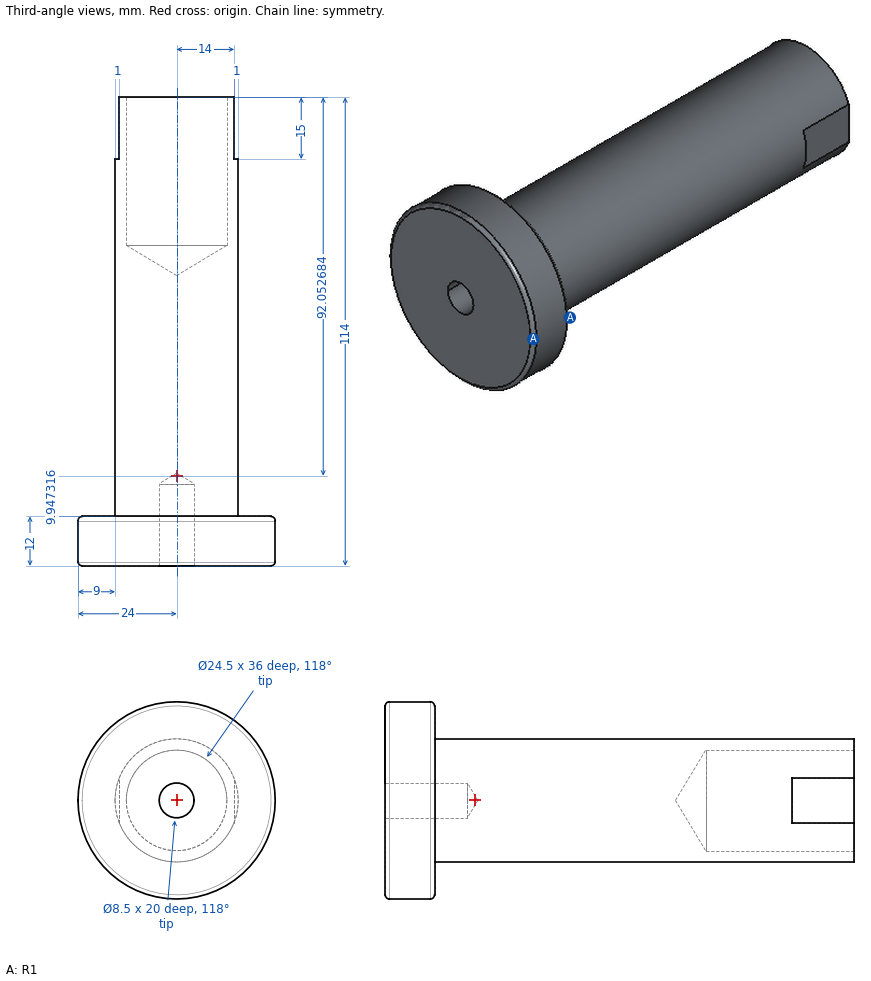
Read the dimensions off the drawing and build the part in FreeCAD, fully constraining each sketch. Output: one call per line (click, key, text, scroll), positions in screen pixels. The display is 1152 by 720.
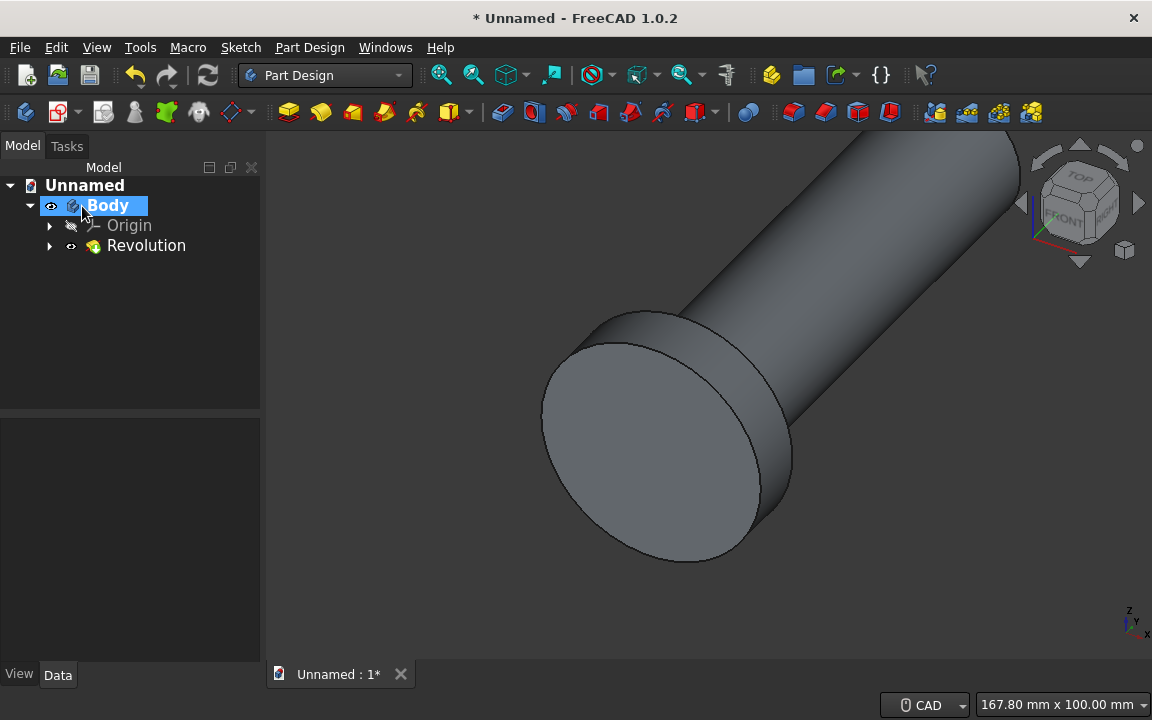
key(v)
key(f)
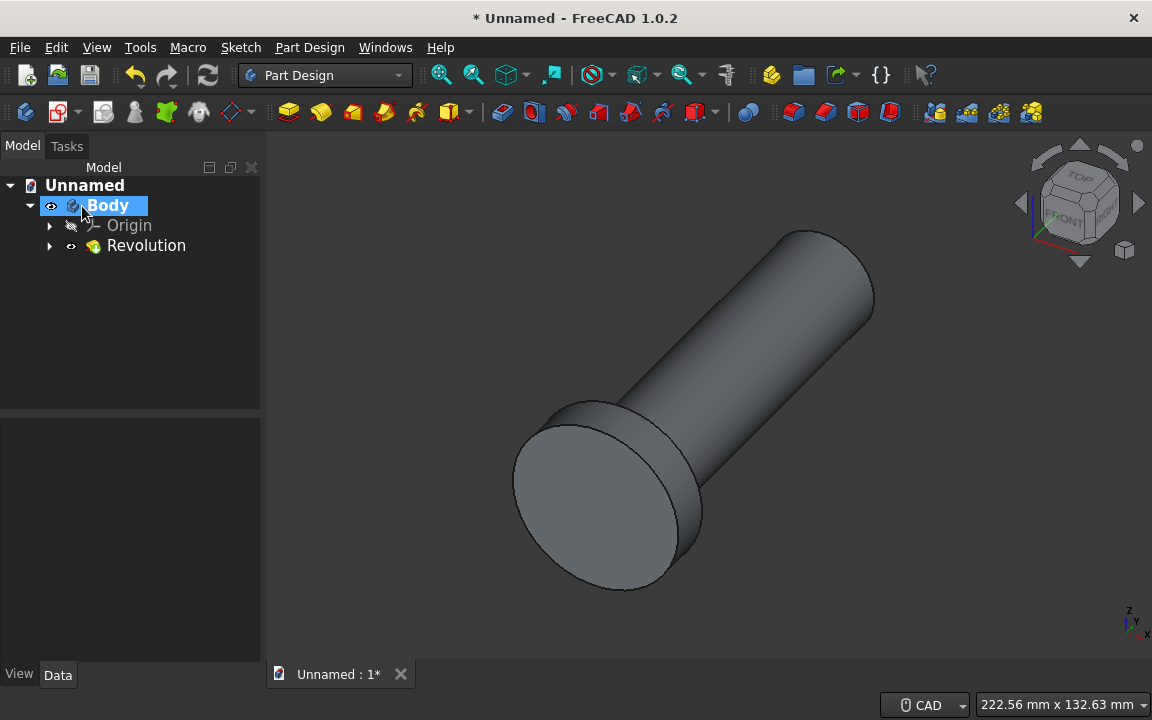
click(58, 112)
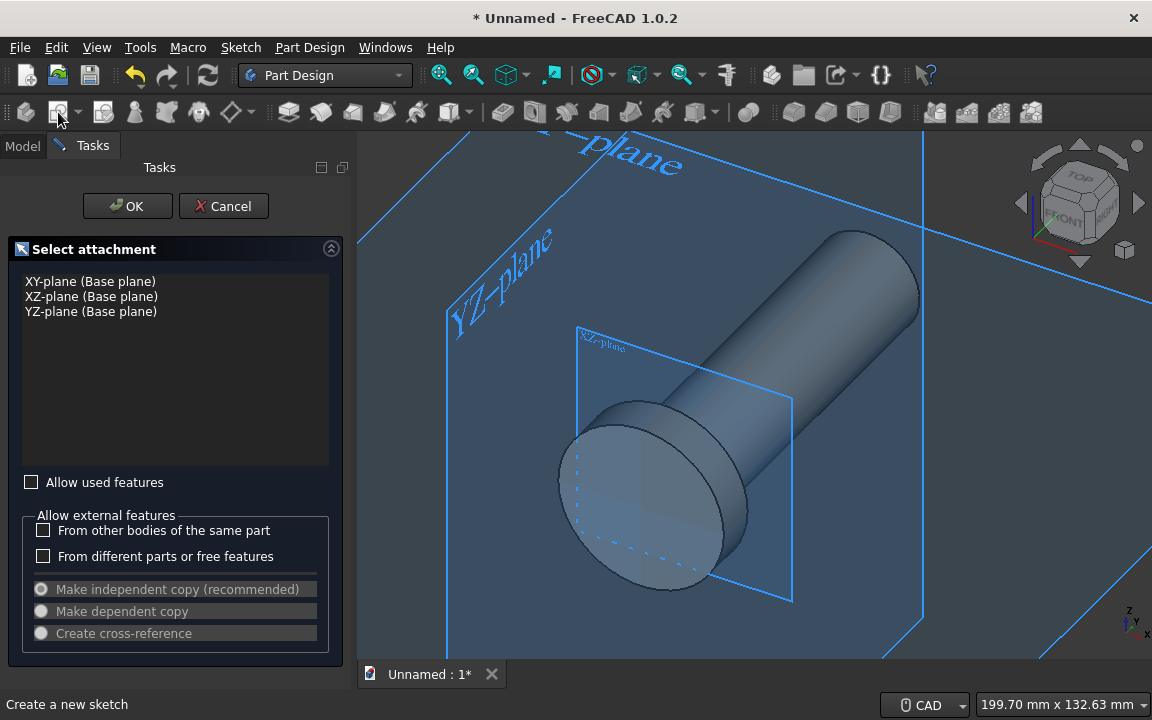
click(82, 282)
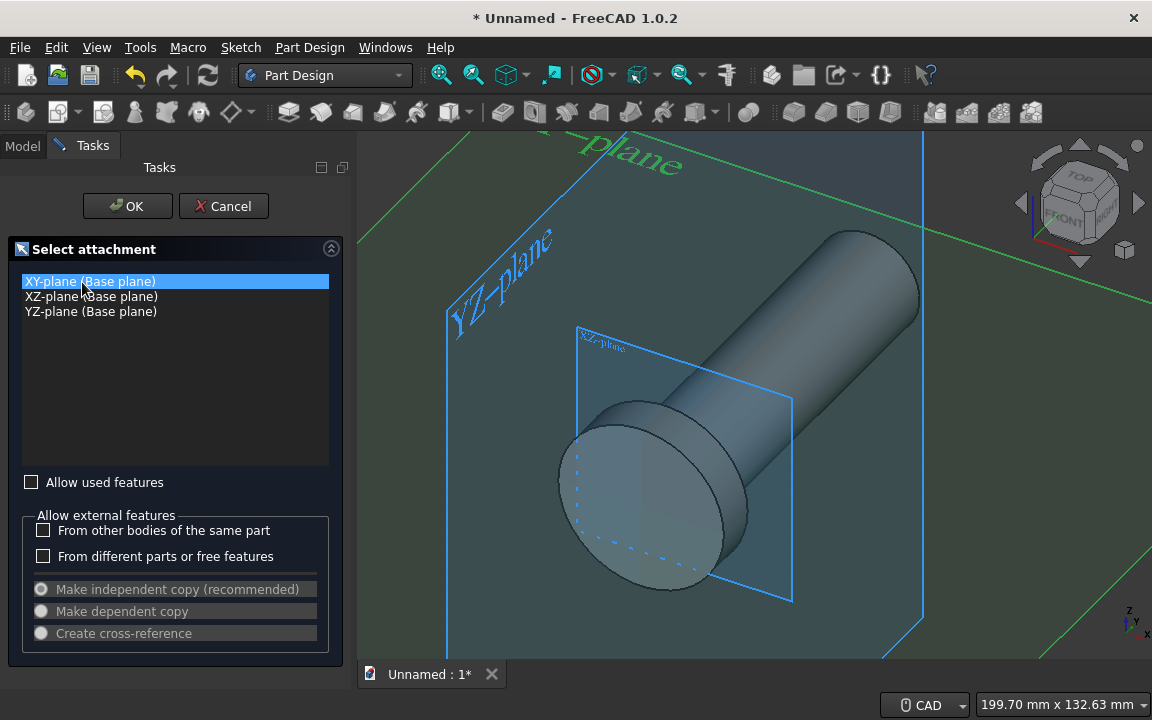
click(128, 206)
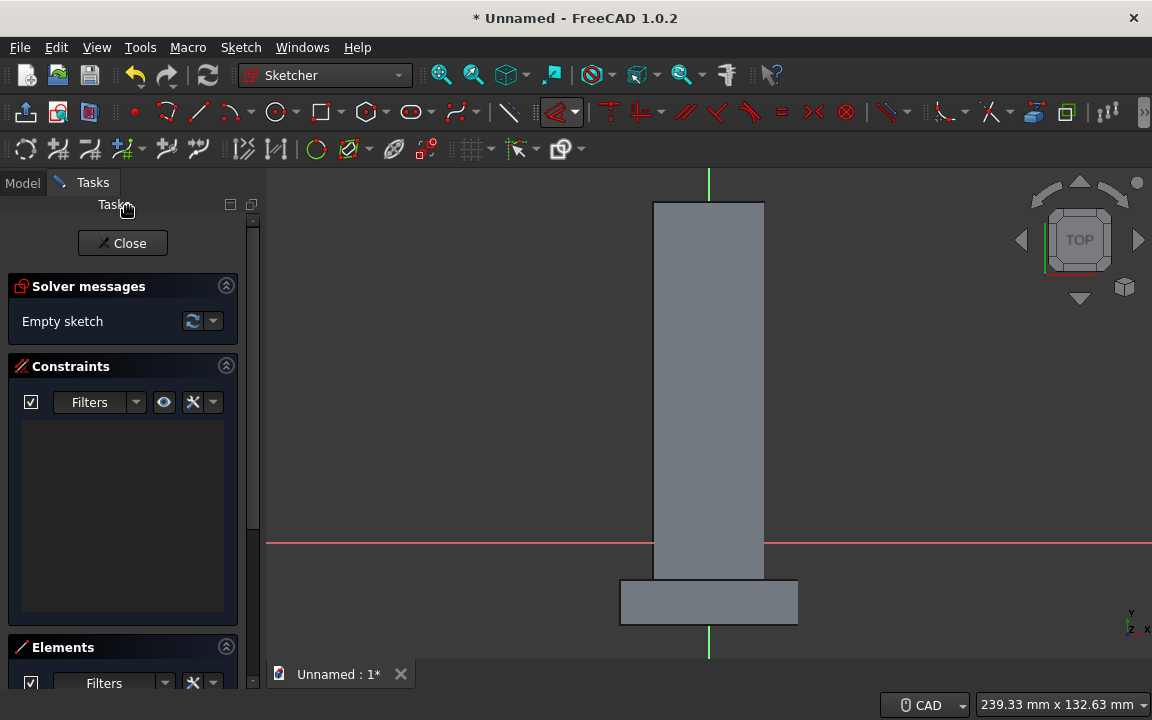
key(q)
key(s)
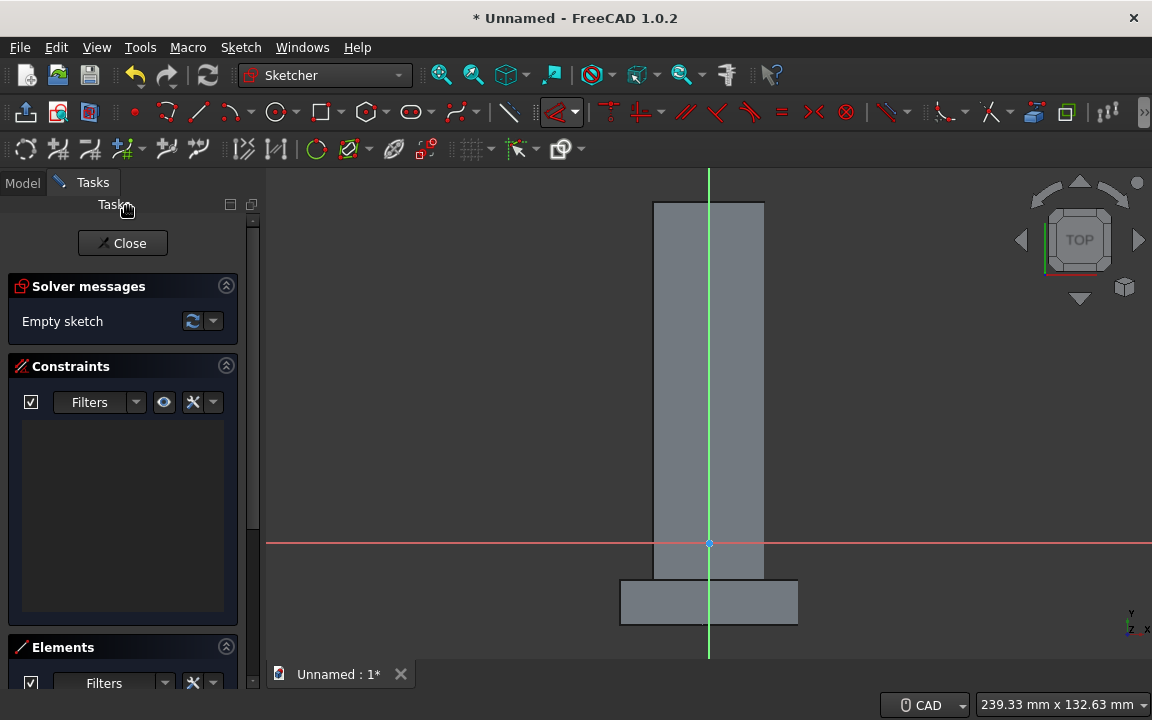
scroll(731, 196, up, 7)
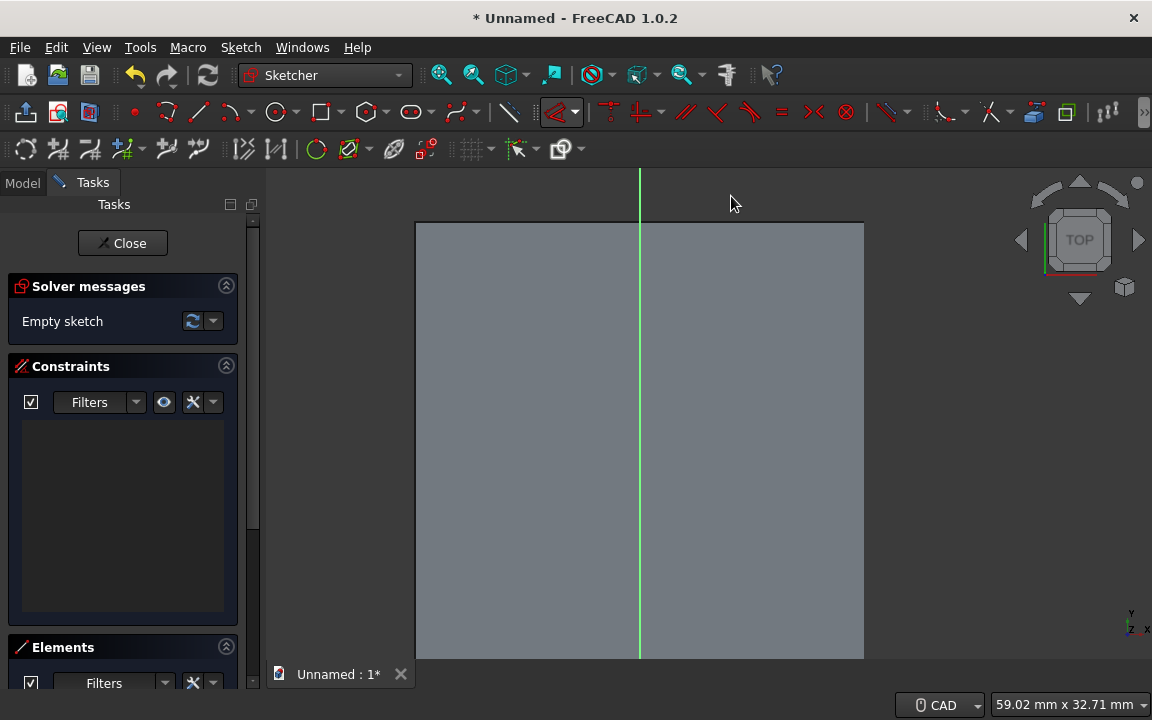
click(322, 112)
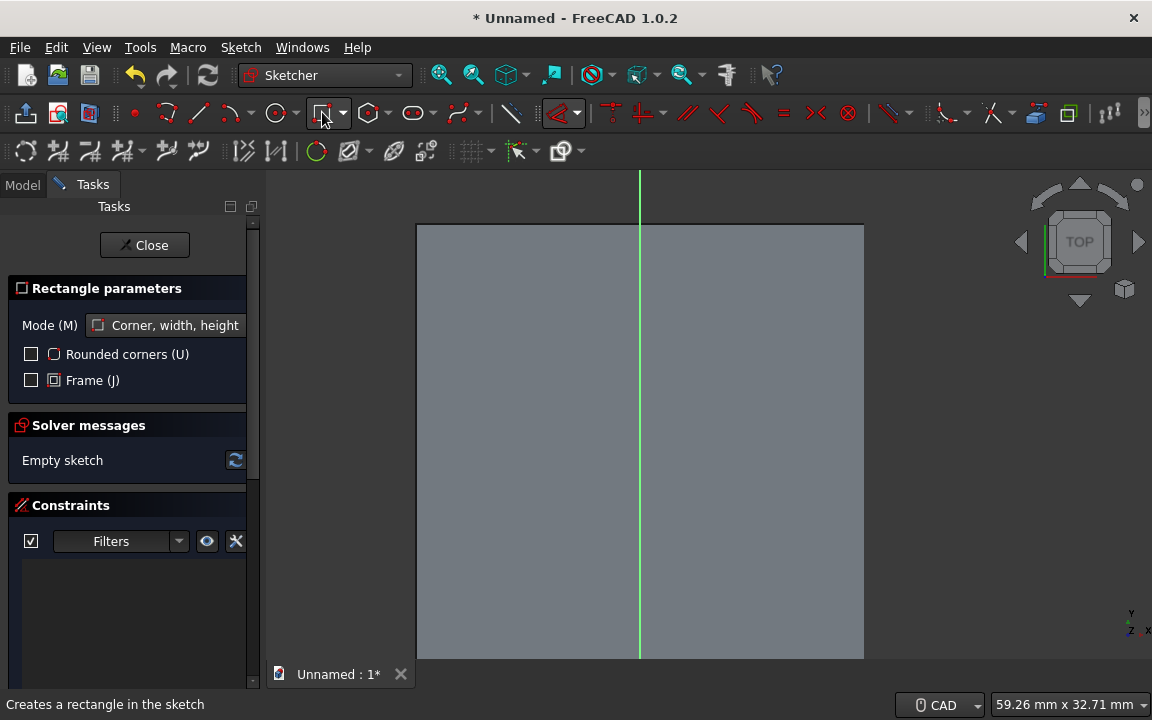
click(850, 224)
move(865, 448)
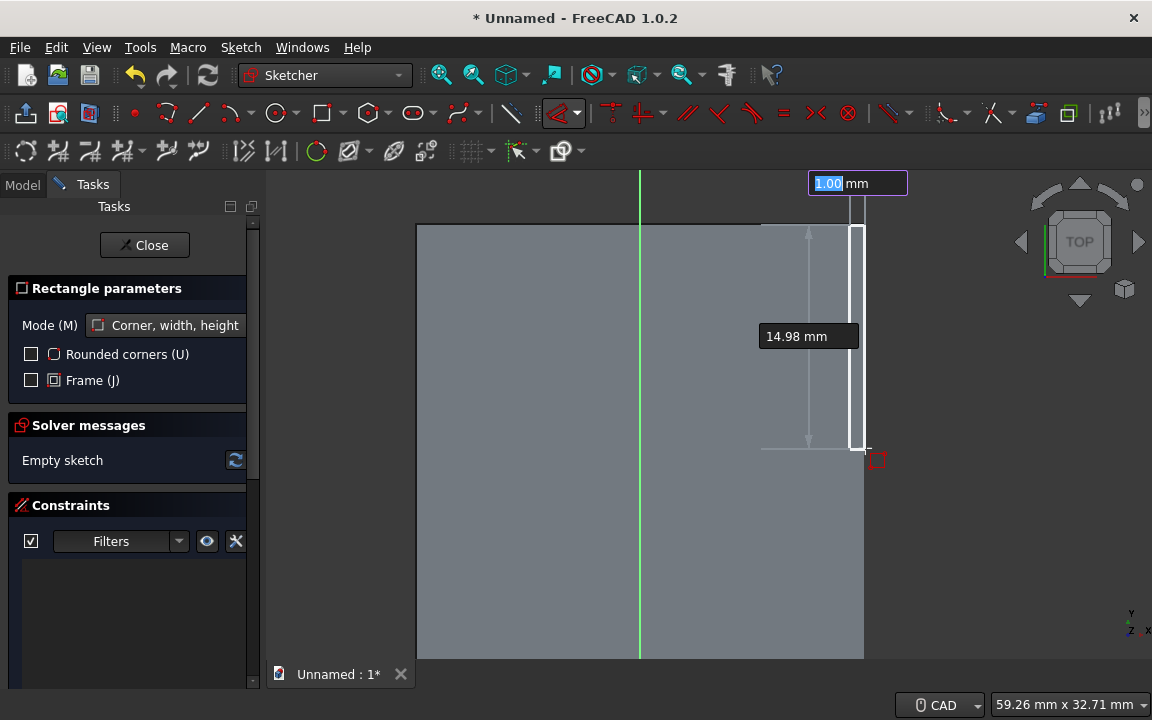
text(1)
key(Tab)
text(15)
key(Return)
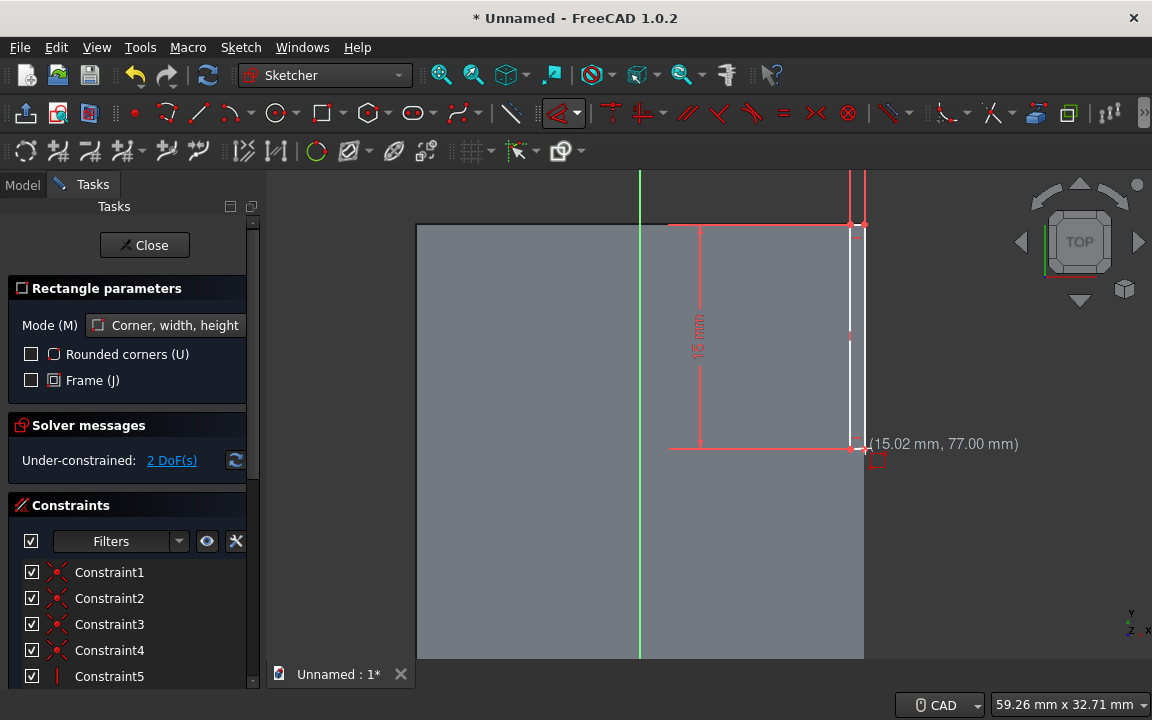
click(416, 224)
move(431, 448)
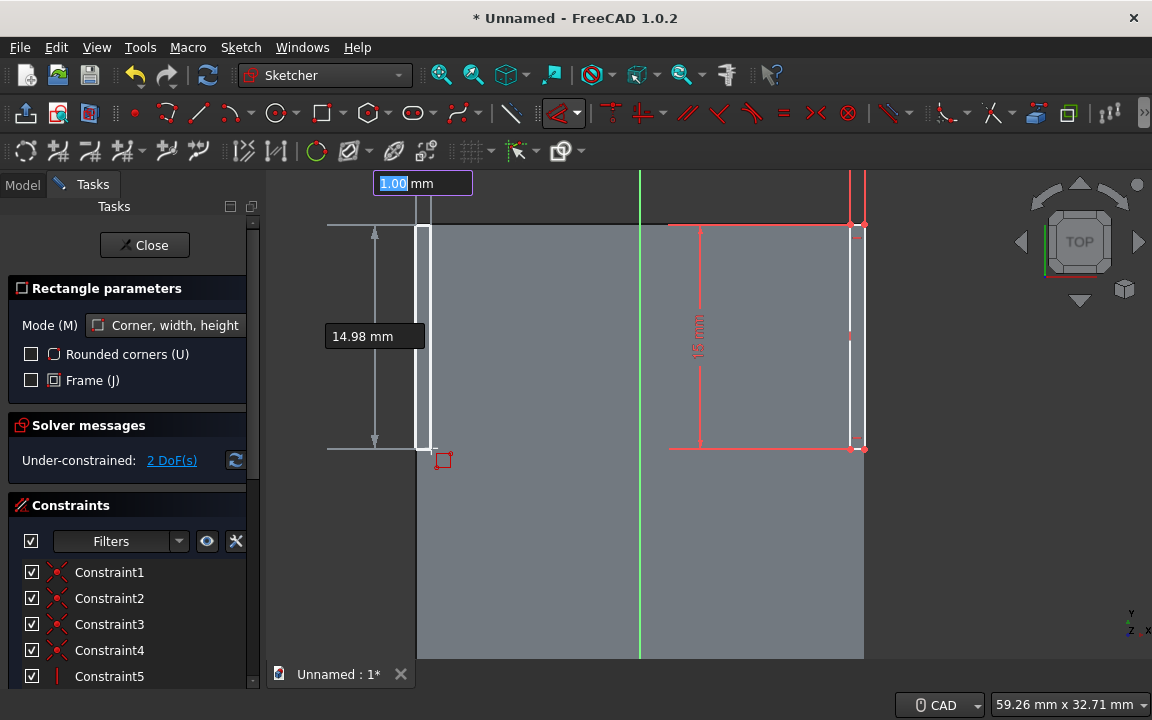
text(1)
key(Tab)
text(15)
key(Return)
key(Escape)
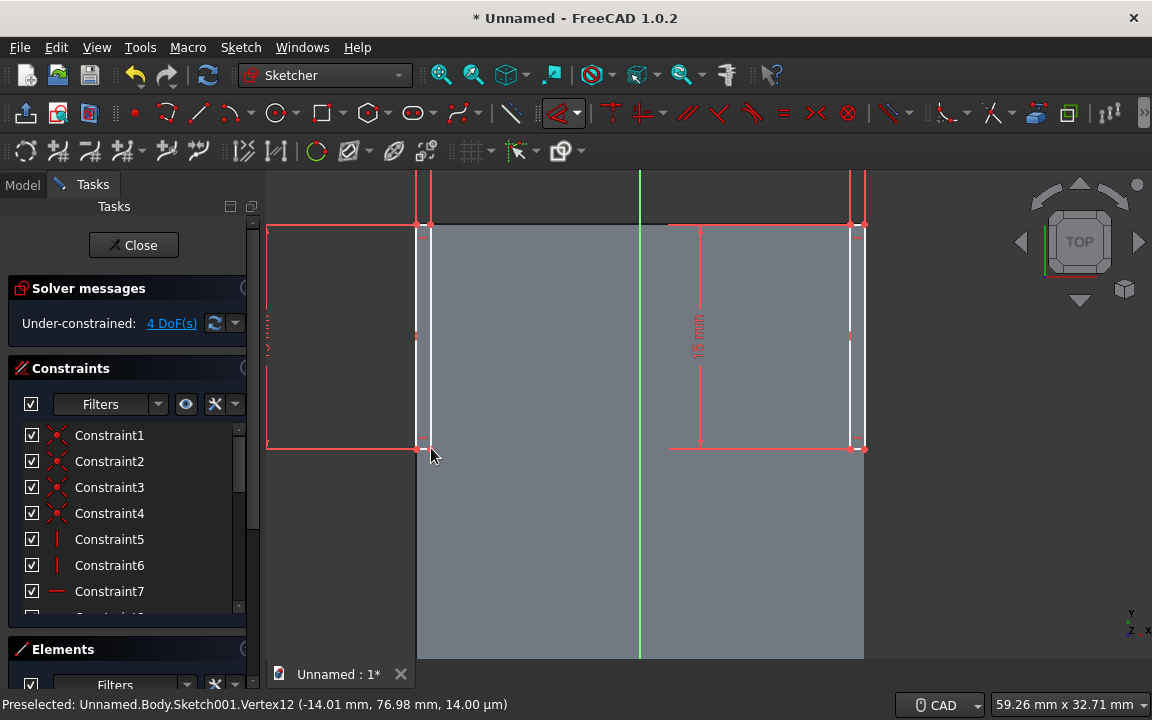
click(865, 225)